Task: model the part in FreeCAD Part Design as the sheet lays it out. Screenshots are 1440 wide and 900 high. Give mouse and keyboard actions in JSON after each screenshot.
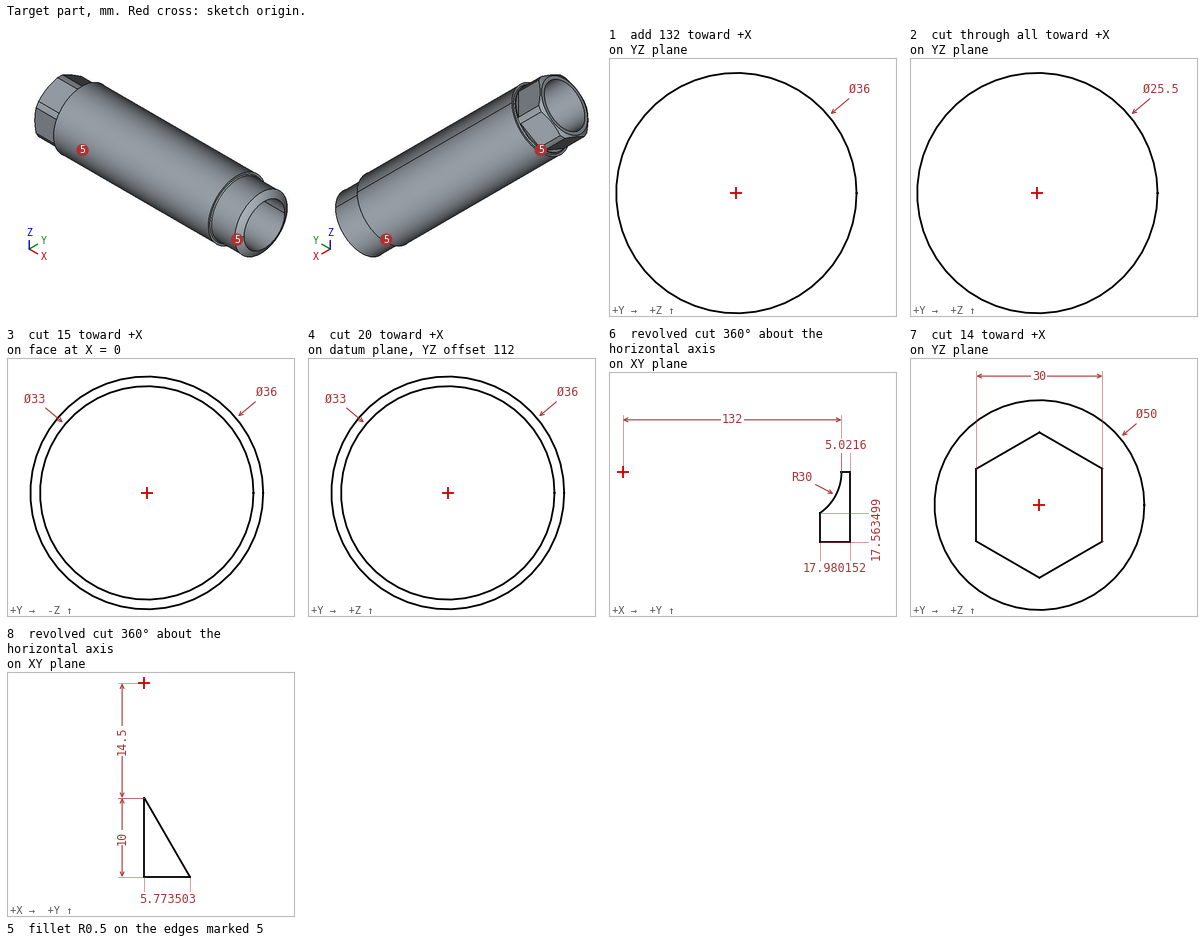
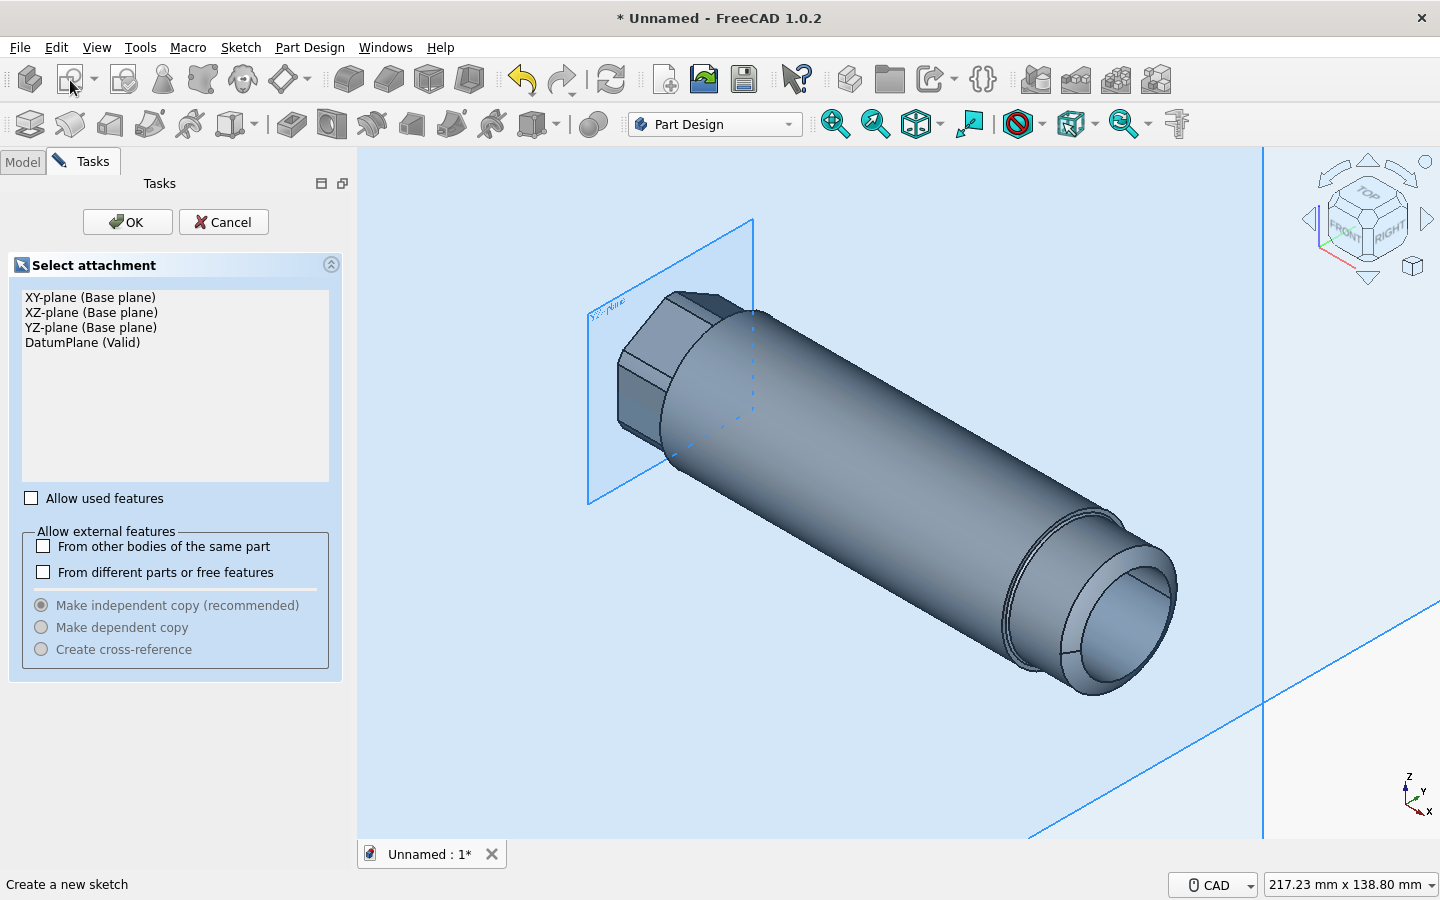
{"action": "left_click", "coordinate": [82, 298]}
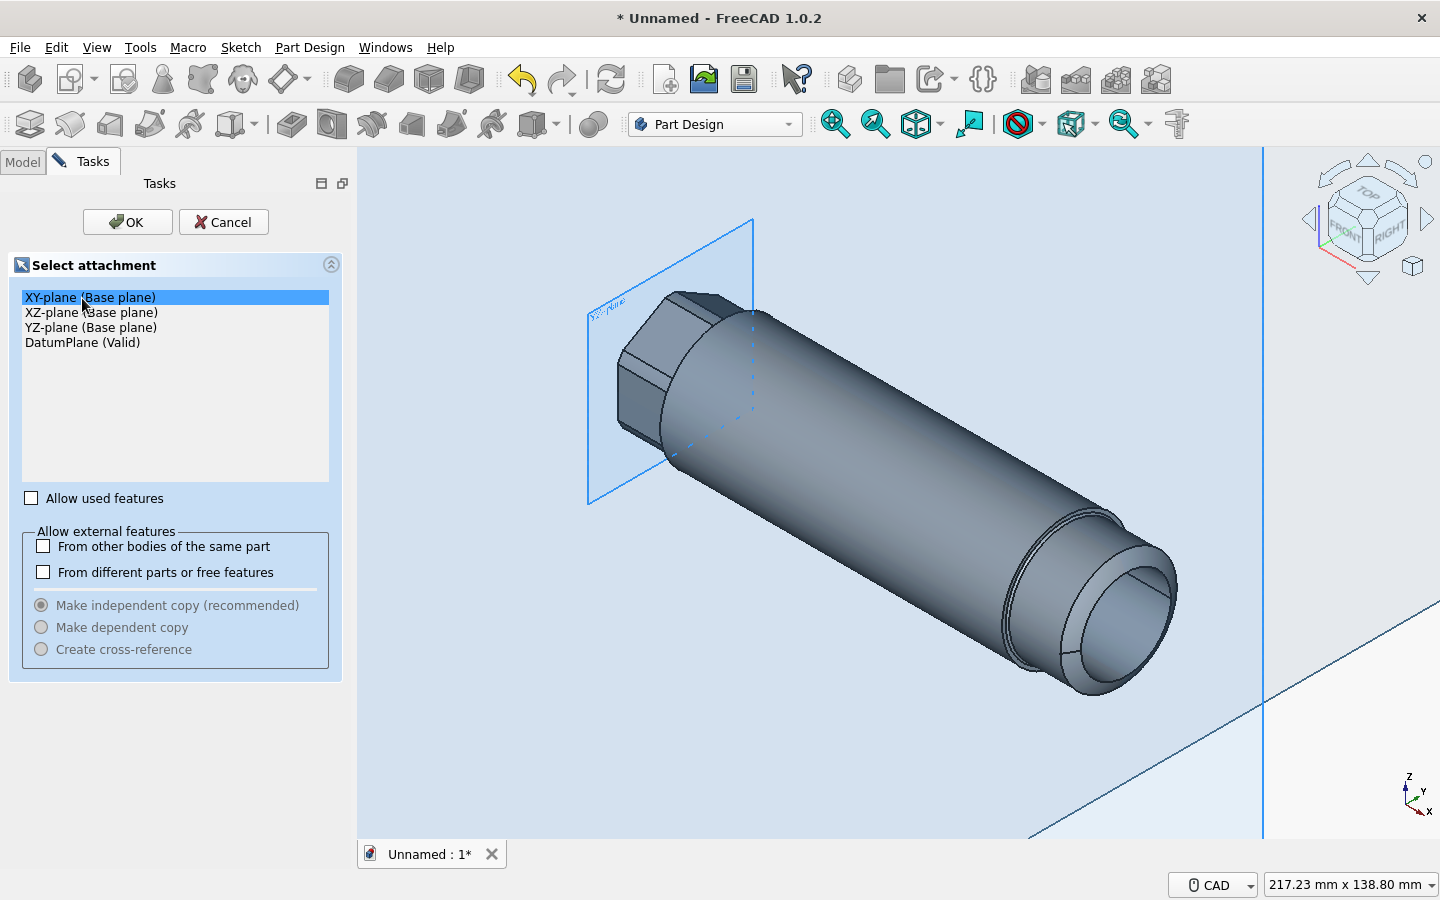
{"action": "left_click", "coordinate": [128, 222]}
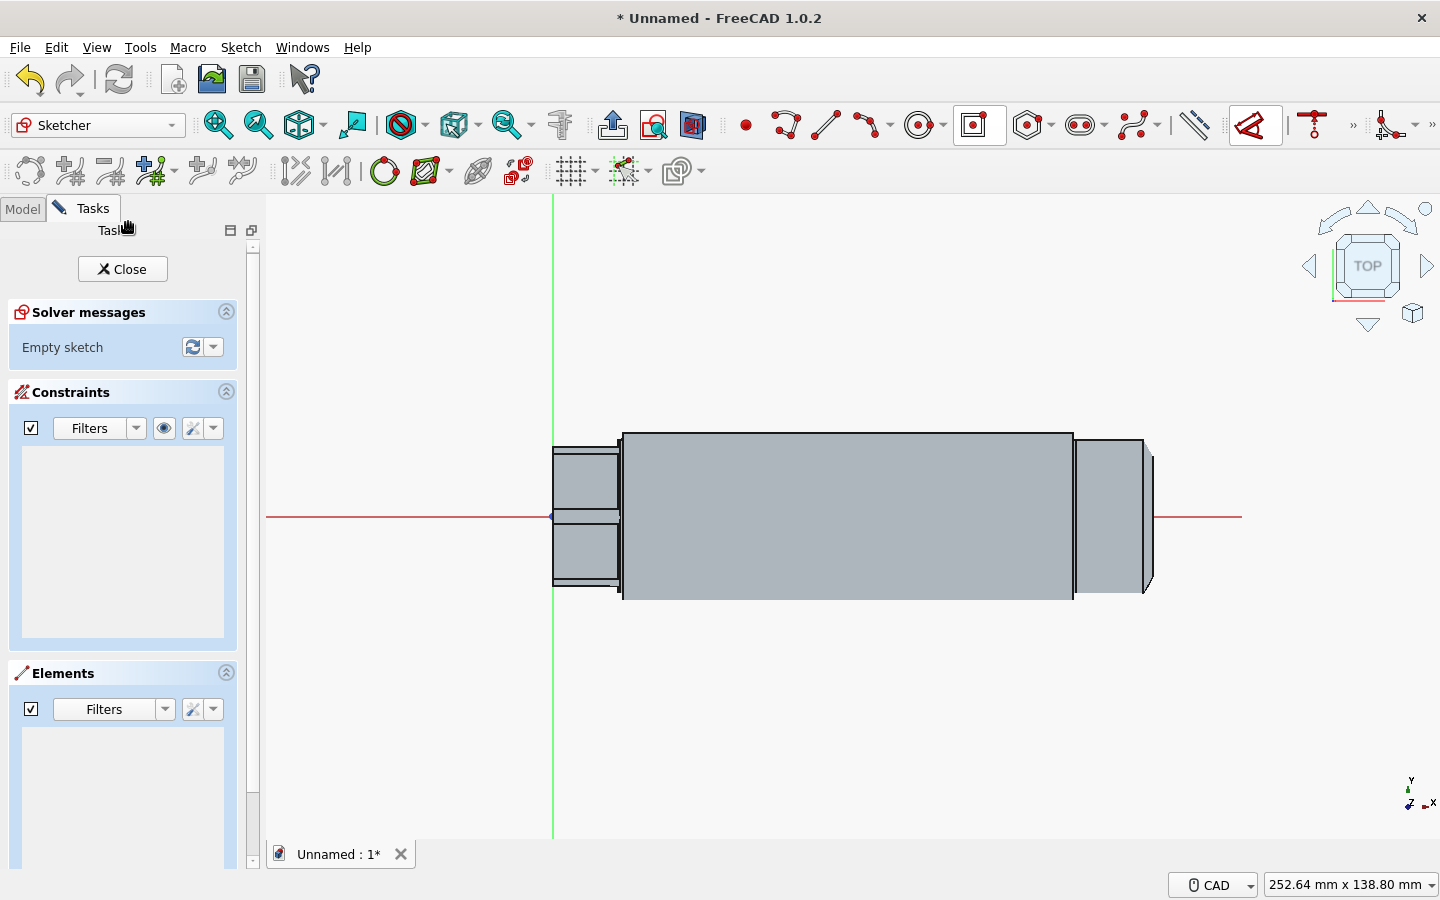
{"action": "key", "text": "q s"}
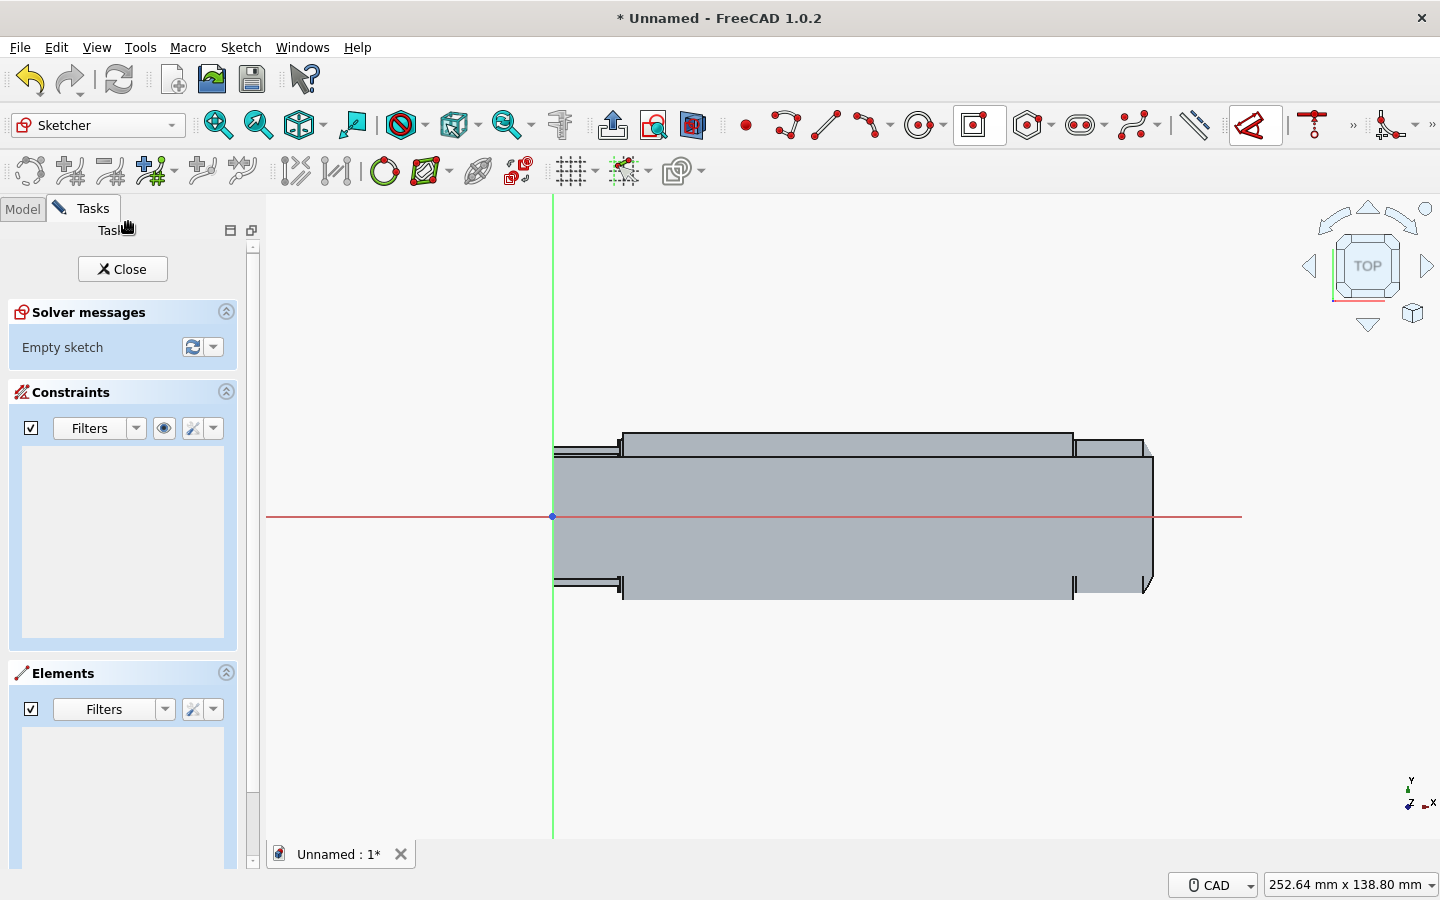
{"action": "scroll", "coordinate": [472, 598], "scroll_direction": "up", "scroll_amount": 6}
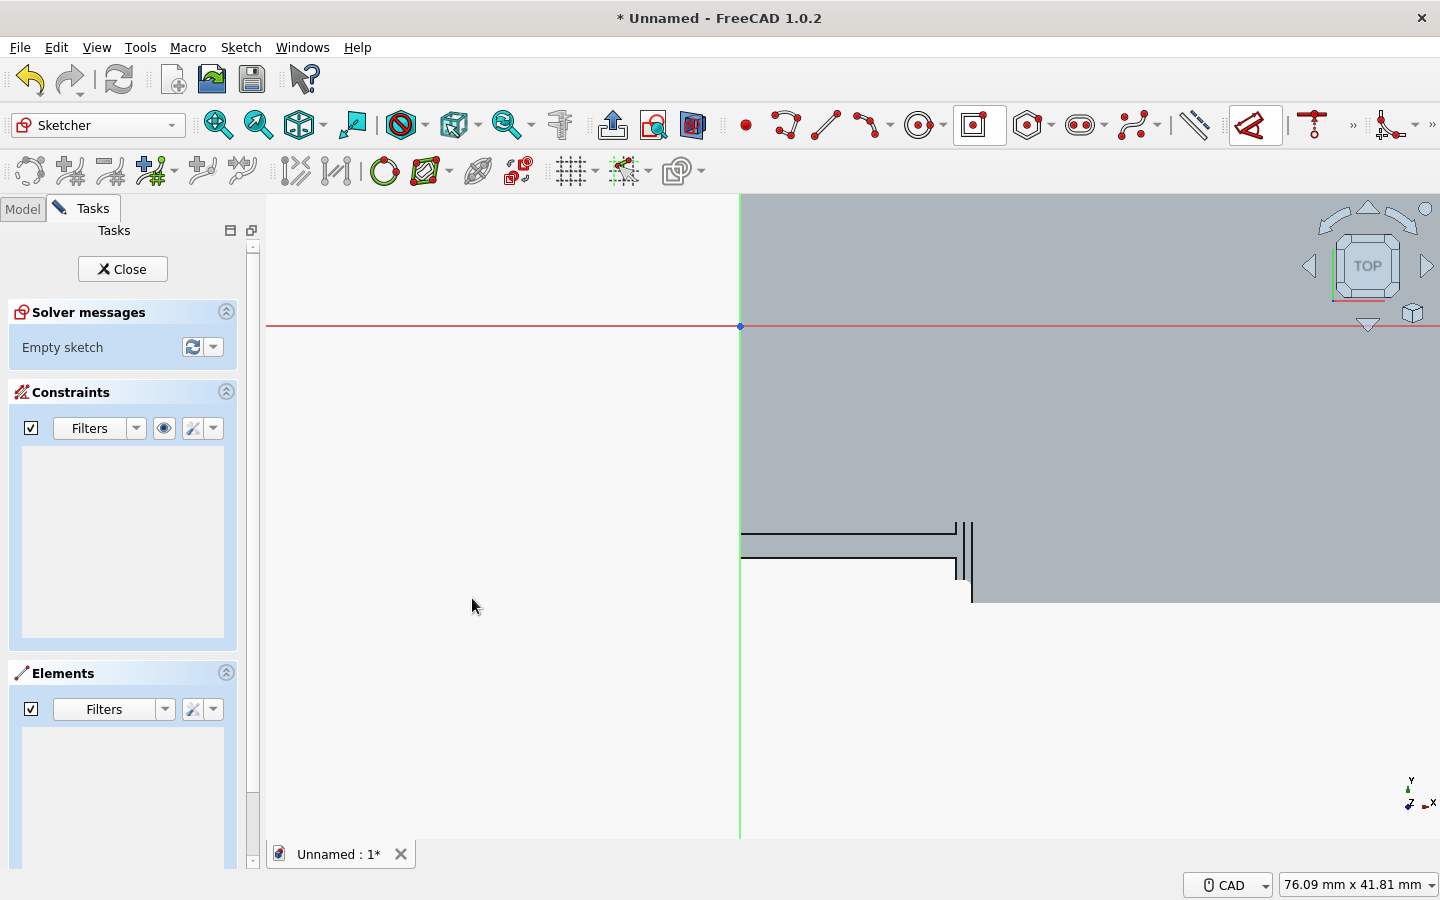
{"action": "left_click", "coordinate": [786, 126]}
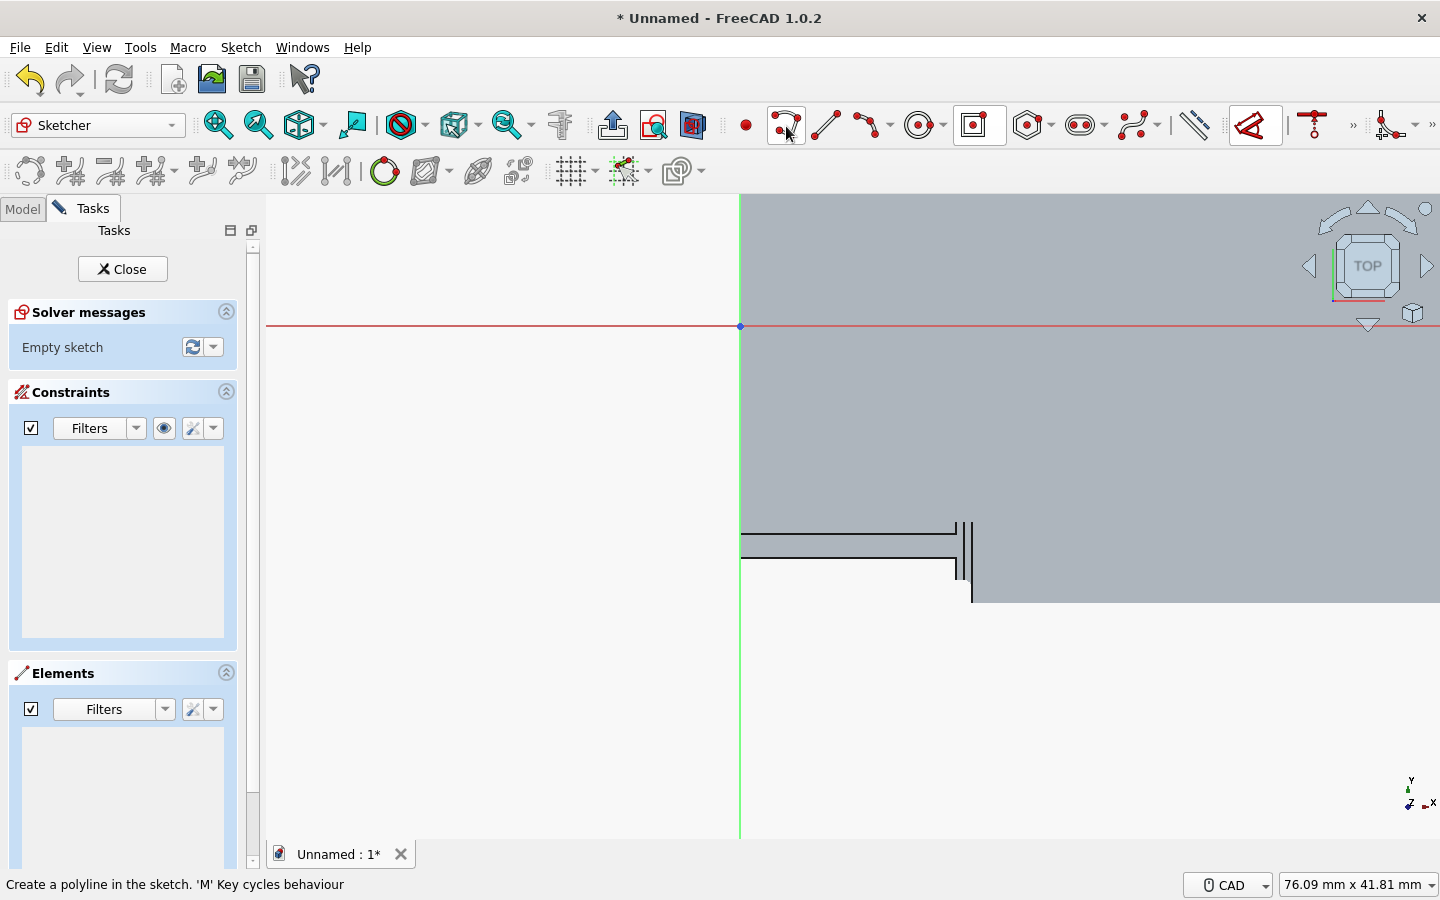
{"action": "left_click", "coordinate": [740, 550]}
{"action": "left_click", "coordinate": [749, 704]}
{"action": "left_click", "coordinate": [829, 704]}
{"action": "left_click", "coordinate": [740, 551]}
{"action": "key", "text": "Escape"}
{"action": "key", "text": "Escape"}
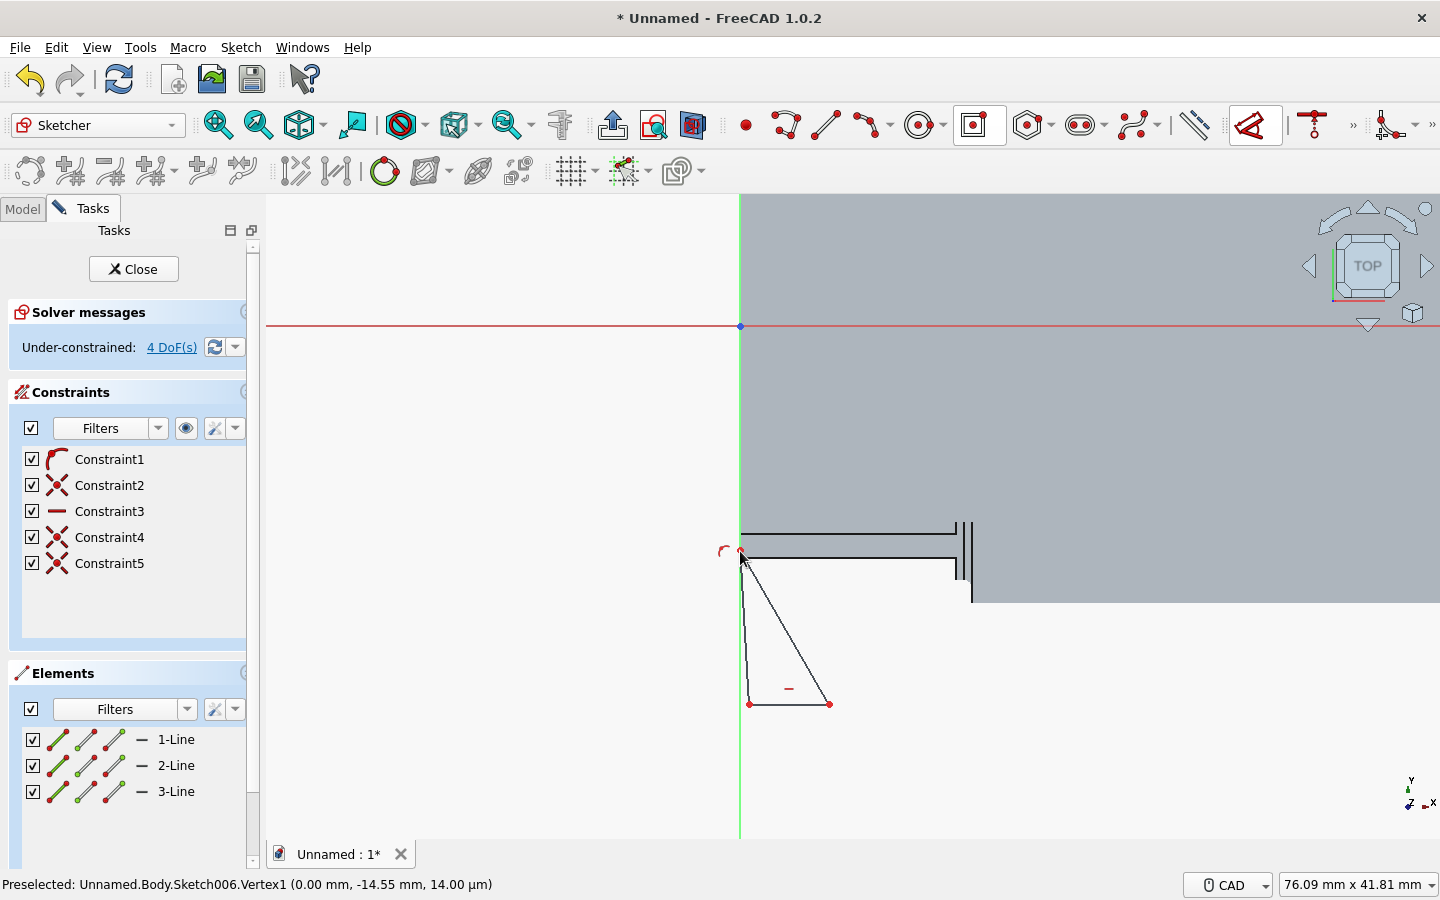
{"action": "left_click", "coordinate": [743, 597]}